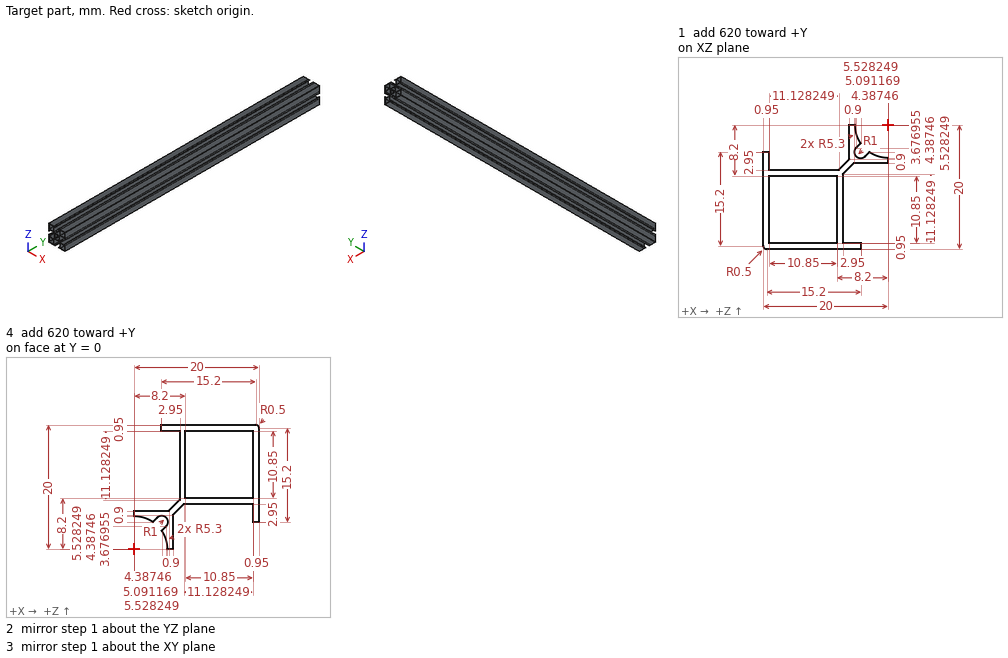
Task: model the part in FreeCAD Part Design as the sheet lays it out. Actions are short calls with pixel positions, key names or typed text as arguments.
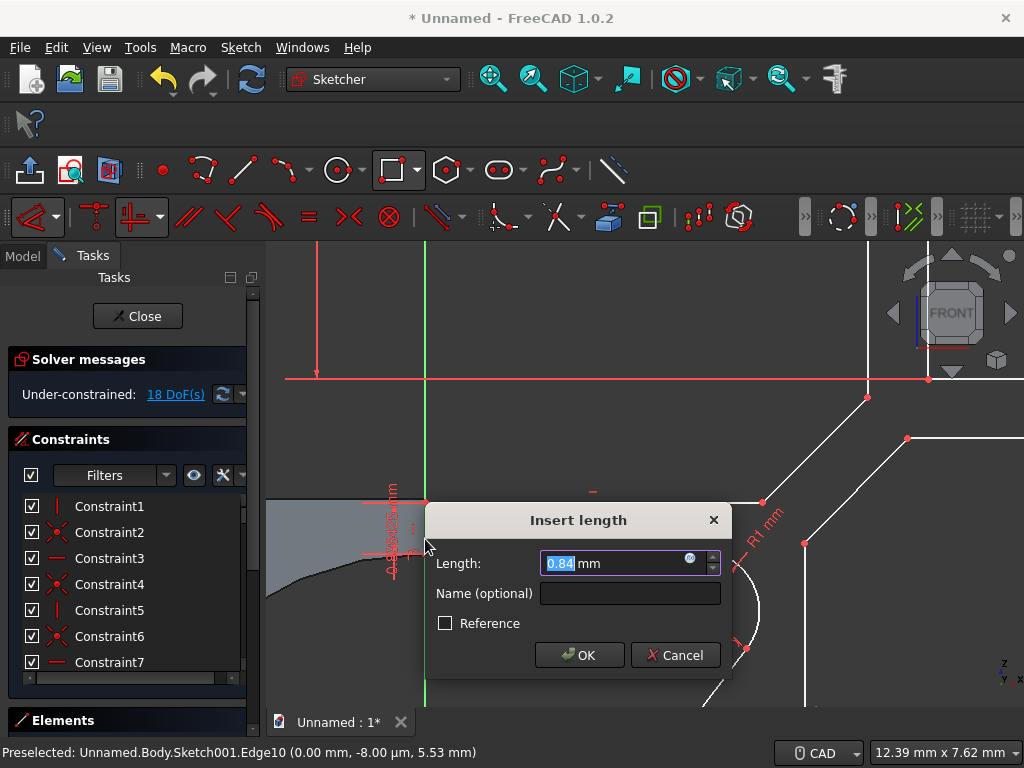
text(0.9)
key(Return)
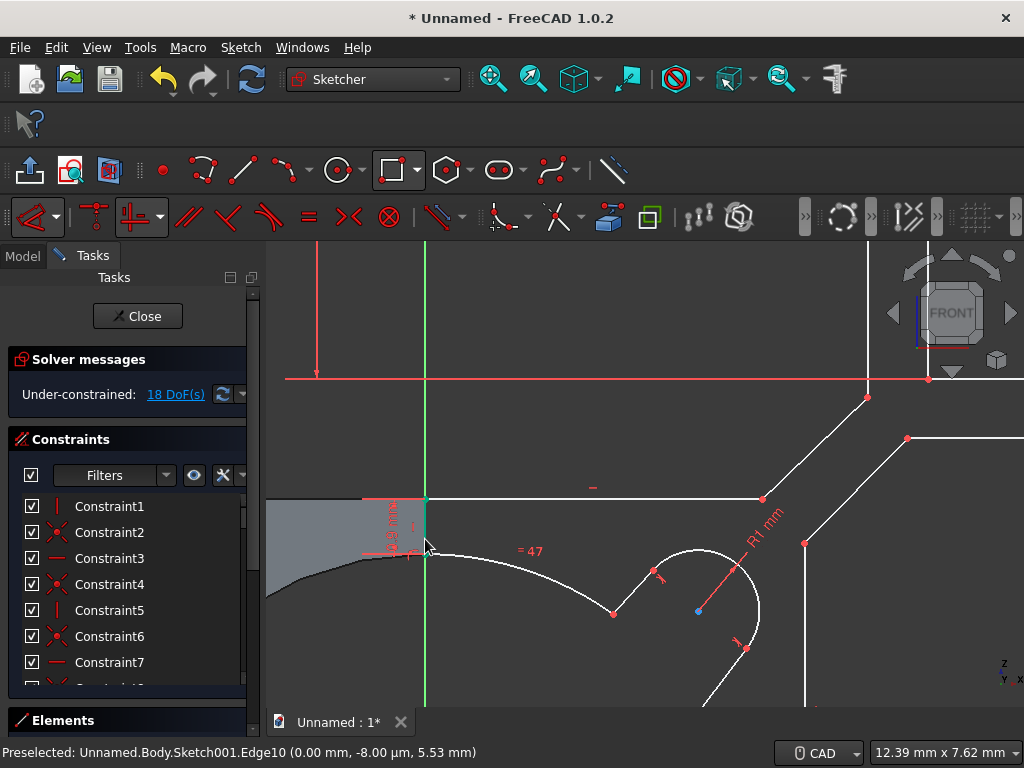
scroll(426, 542, down, 7)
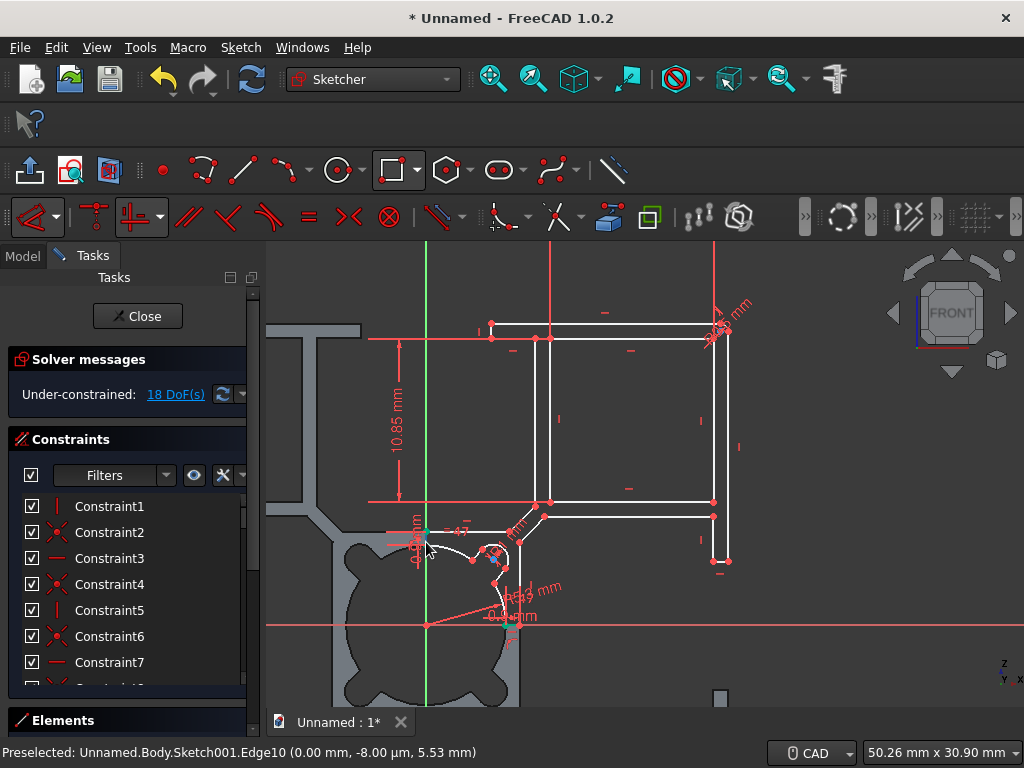
scroll(728, 332, up, 3)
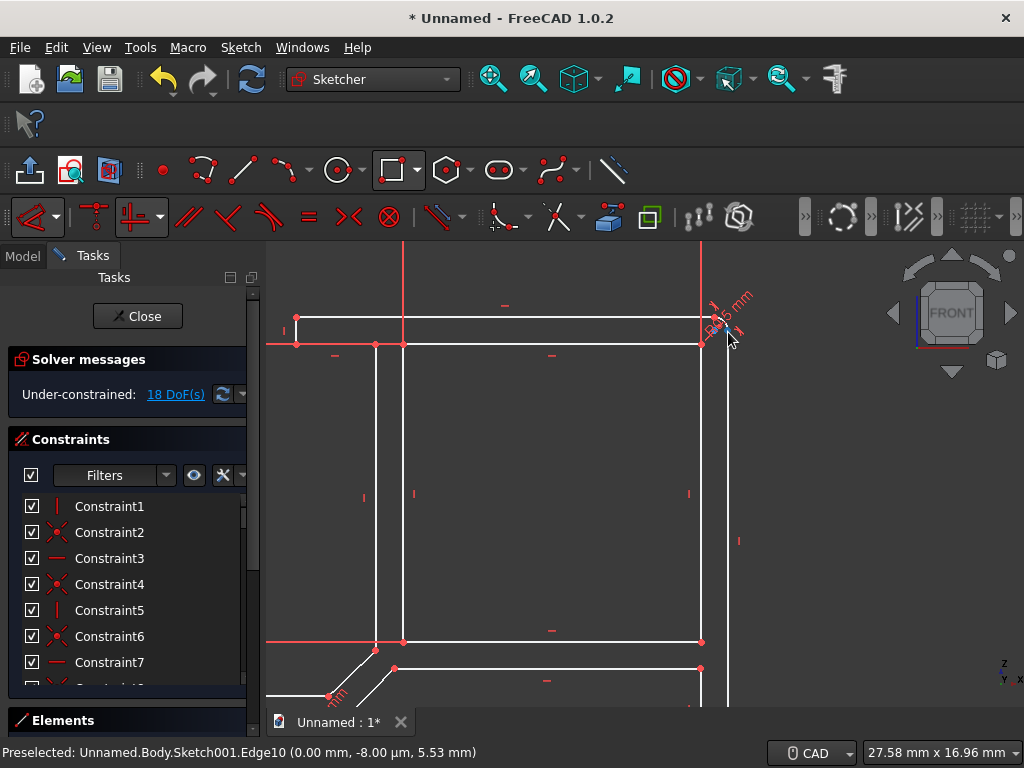
click(728, 331)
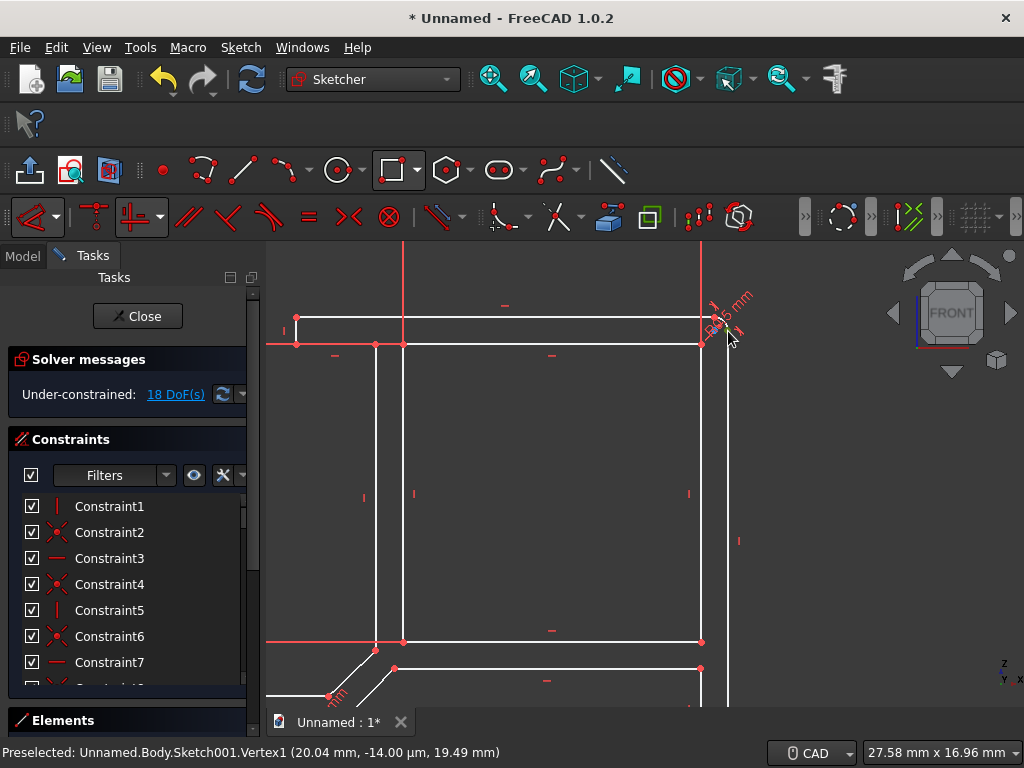
click(58, 218)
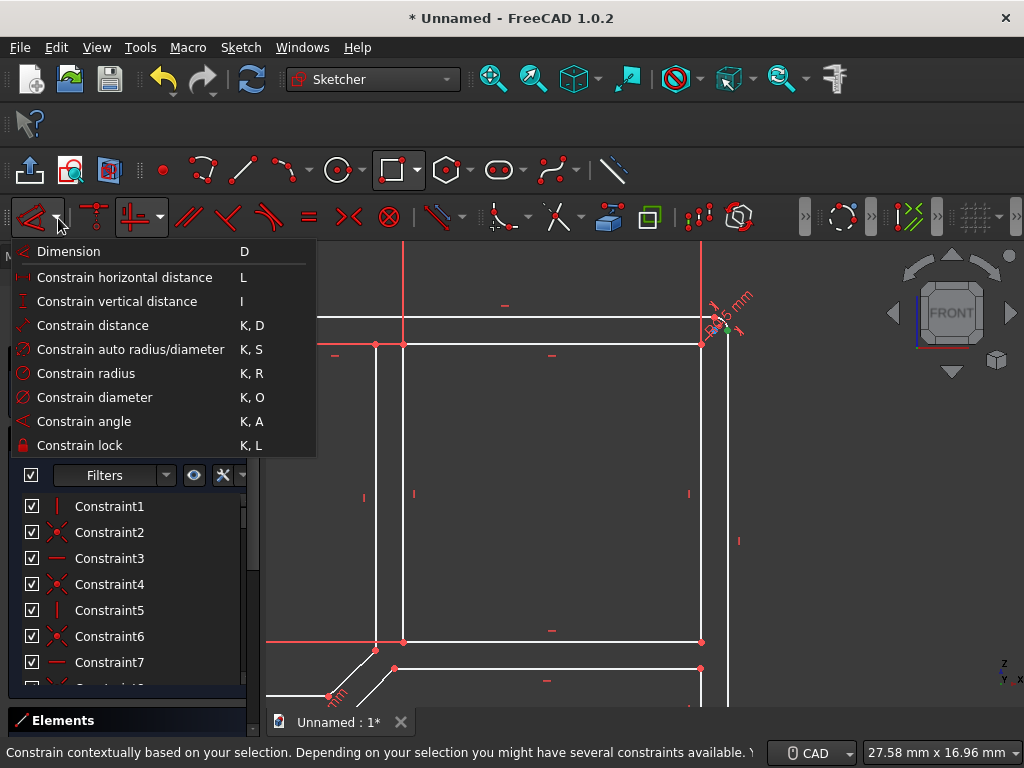
click(164, 277)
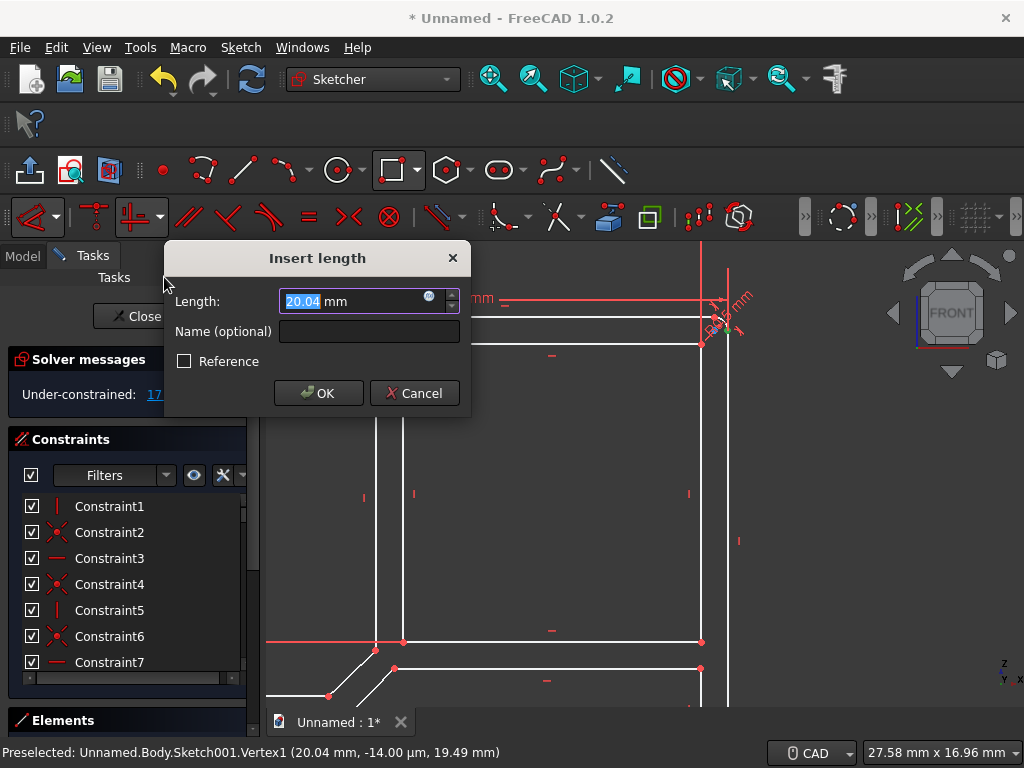
text(20)
key(Return)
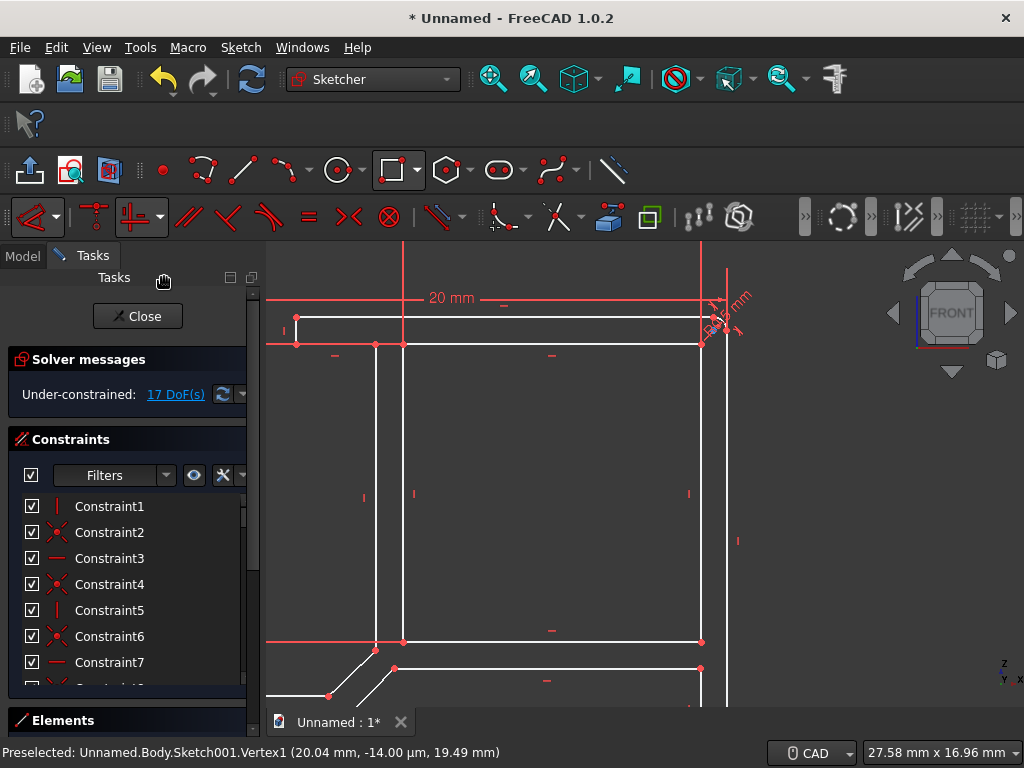
click(296, 317)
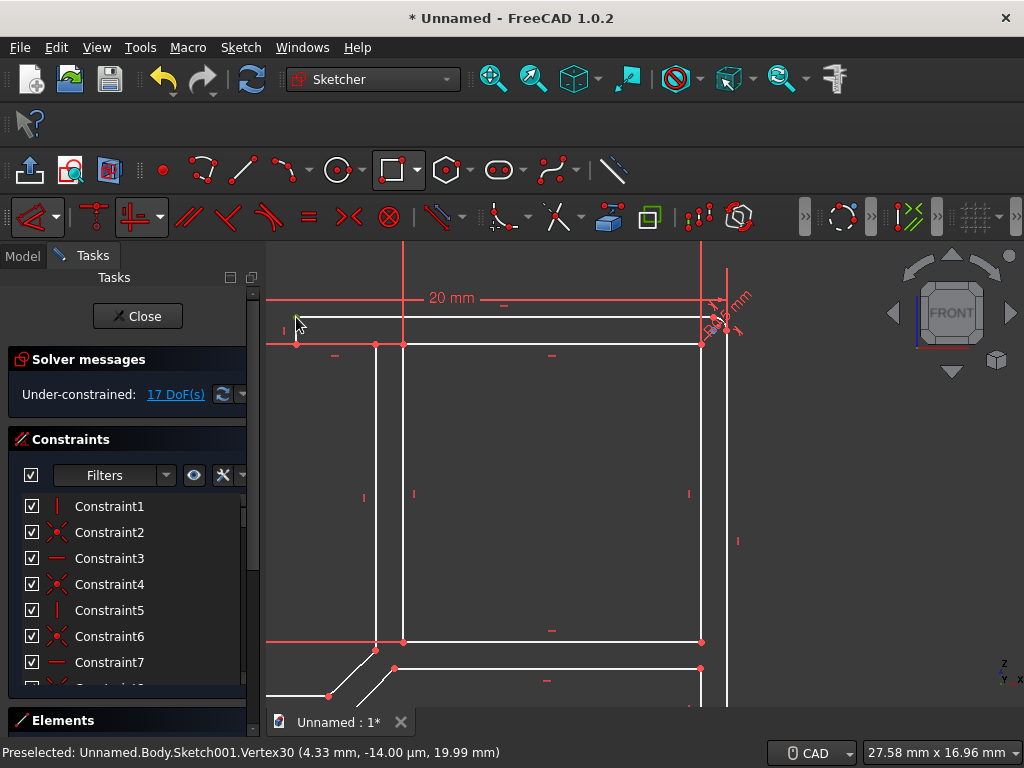
key(i)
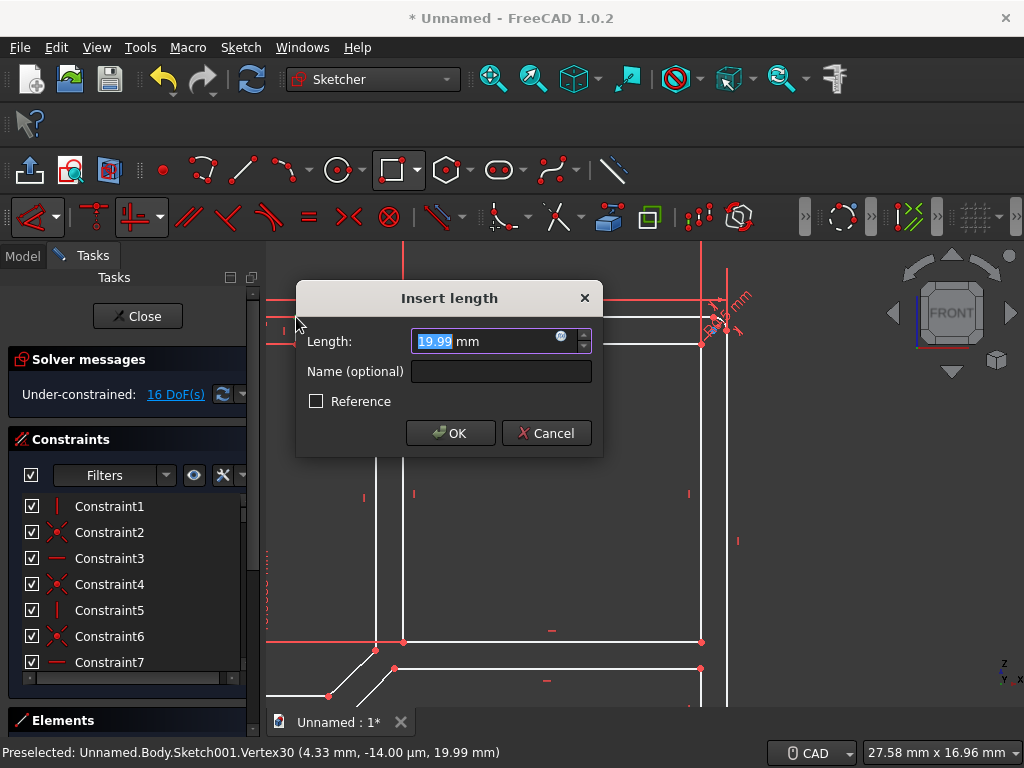
text(20)
key(Return)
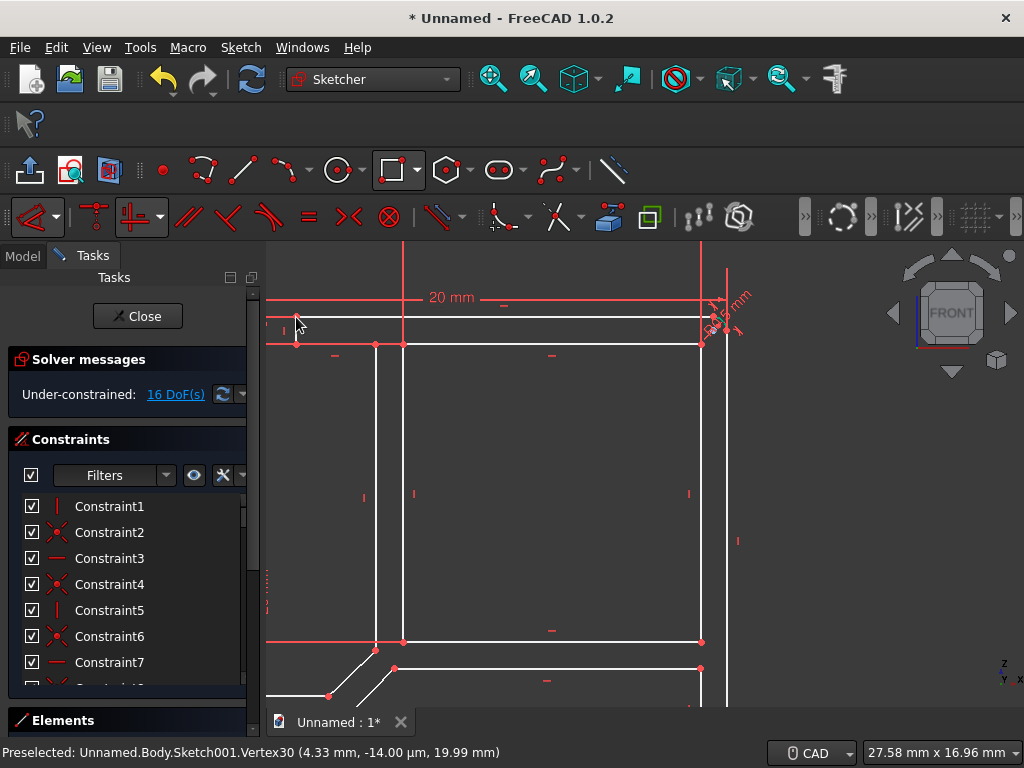
click(727, 457)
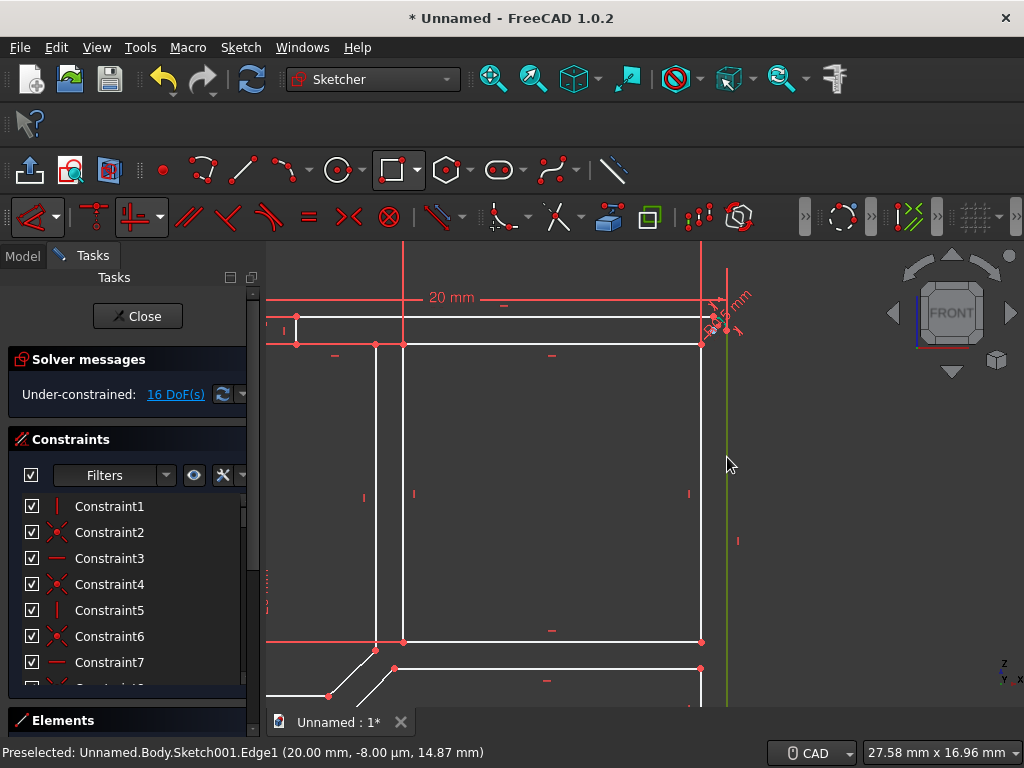
key(i)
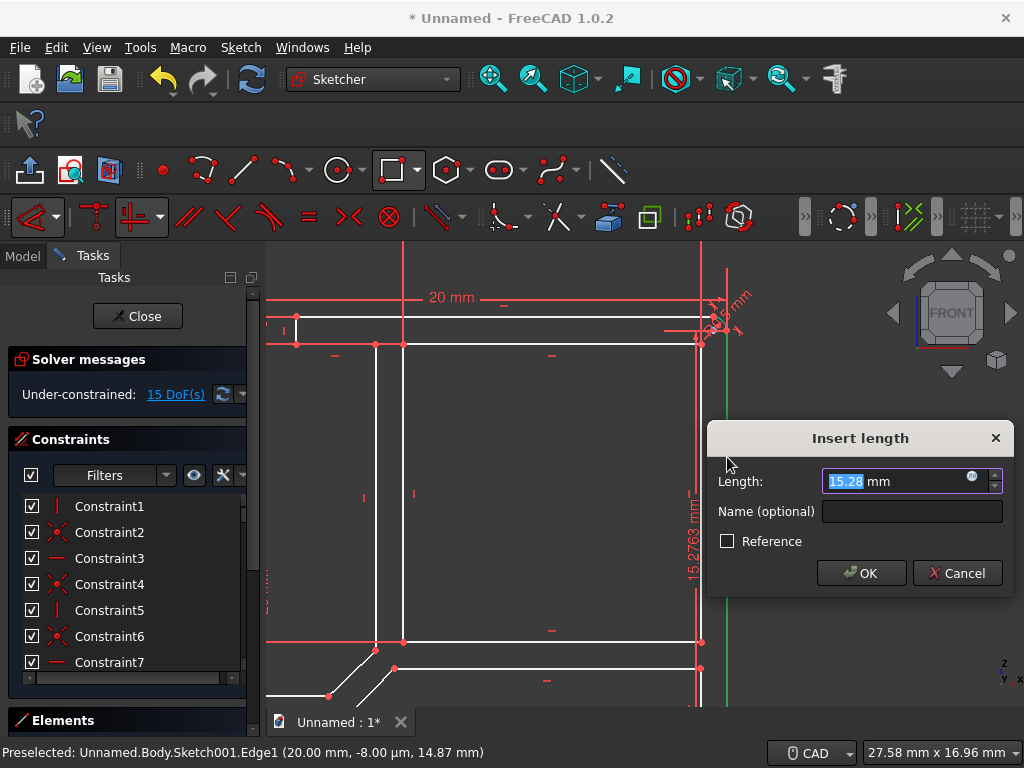
text(15.2)
key(Return)